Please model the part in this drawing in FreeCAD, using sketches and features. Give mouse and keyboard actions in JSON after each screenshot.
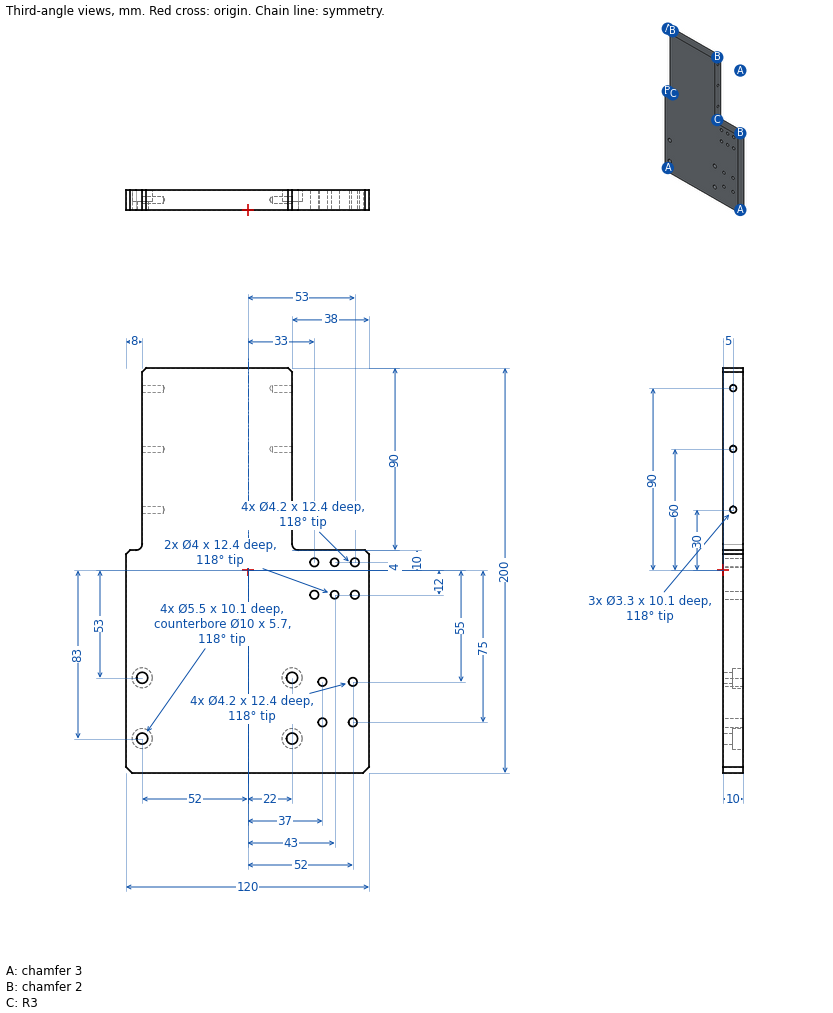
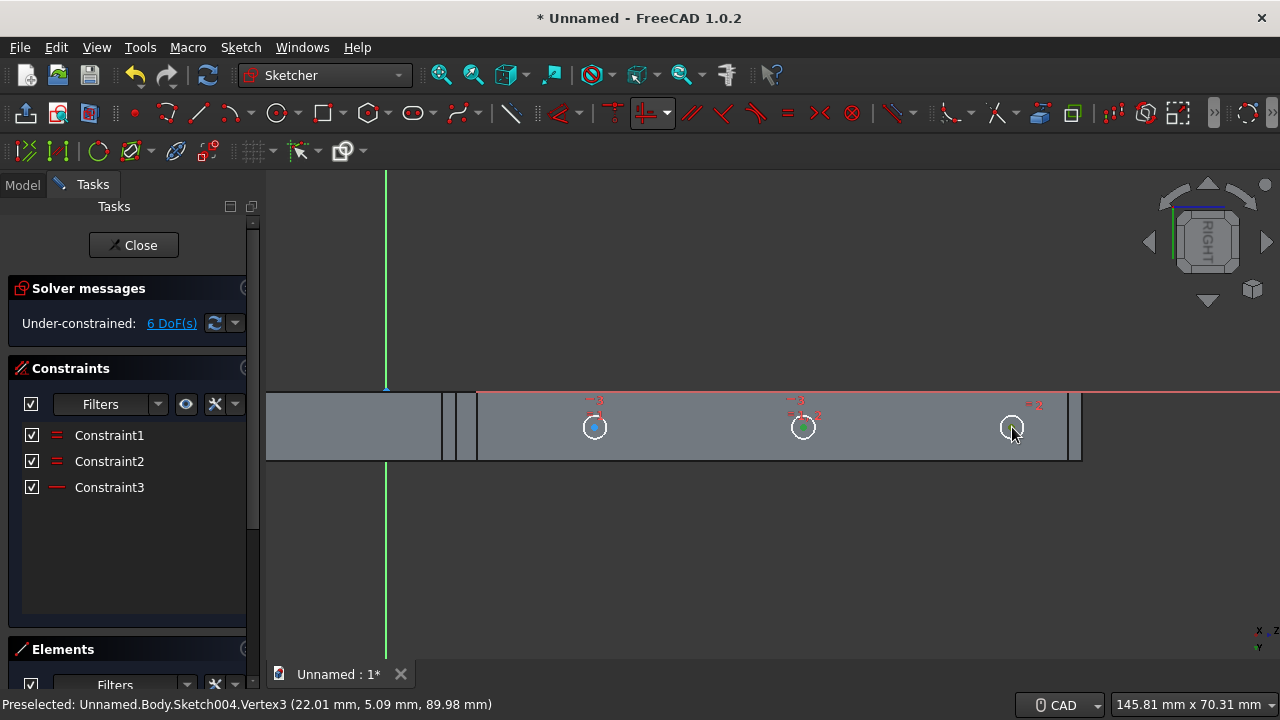
{"action": "key", "text": "h"}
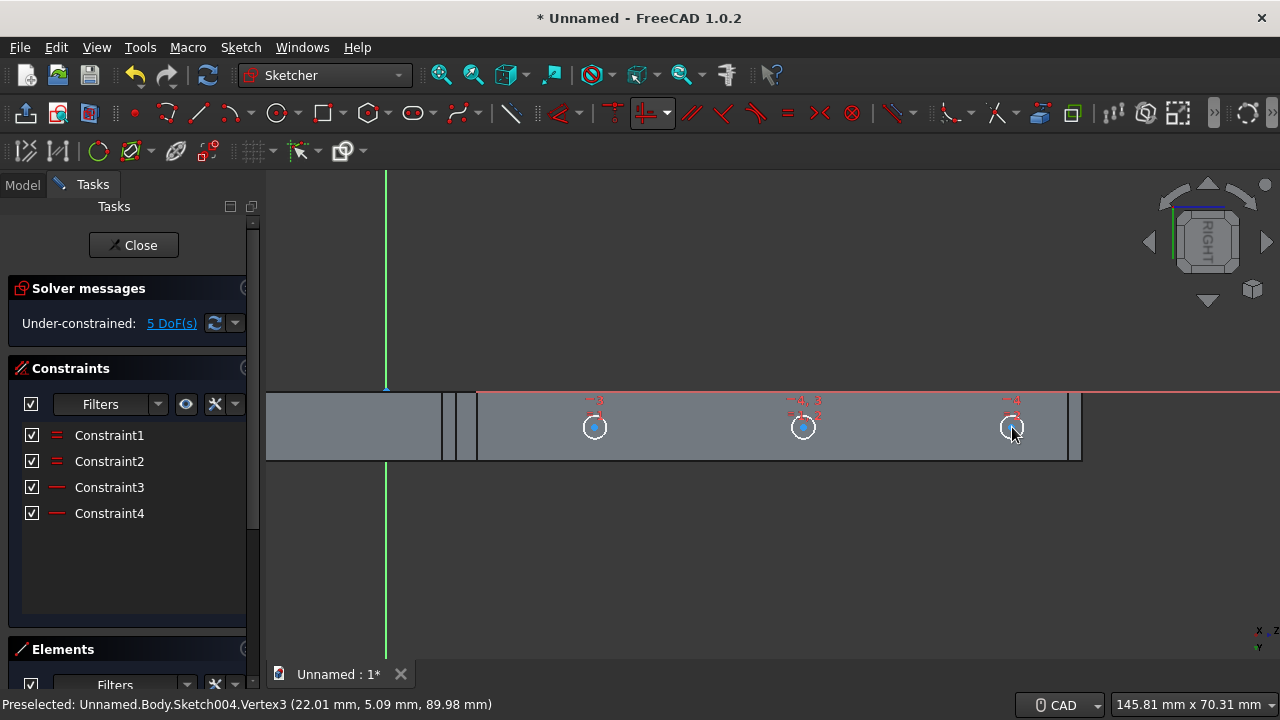
{"action": "left_click", "coordinate": [558, 114]}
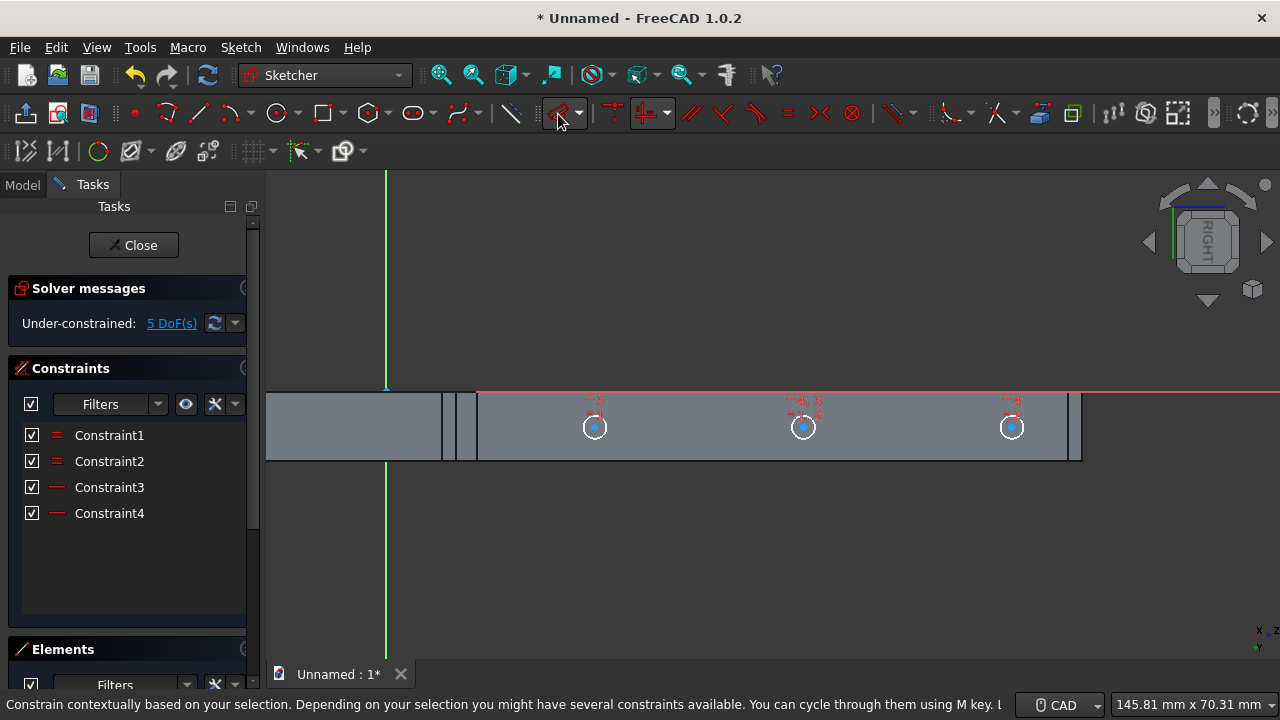
{"action": "scroll", "coordinate": [603, 419], "scroll_direction": "up", "scroll_amount": 3}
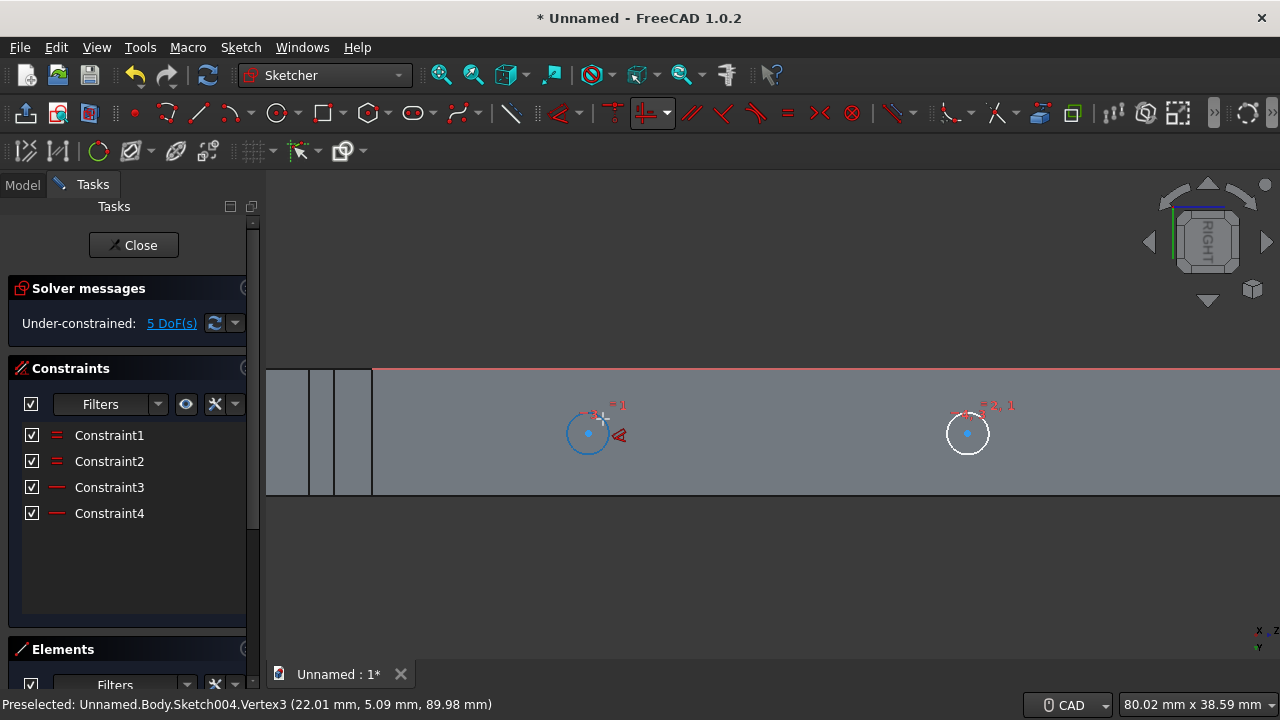
{"action": "left_click", "coordinate": [603, 419]}
{"action": "left_click", "coordinate": [626, 397]}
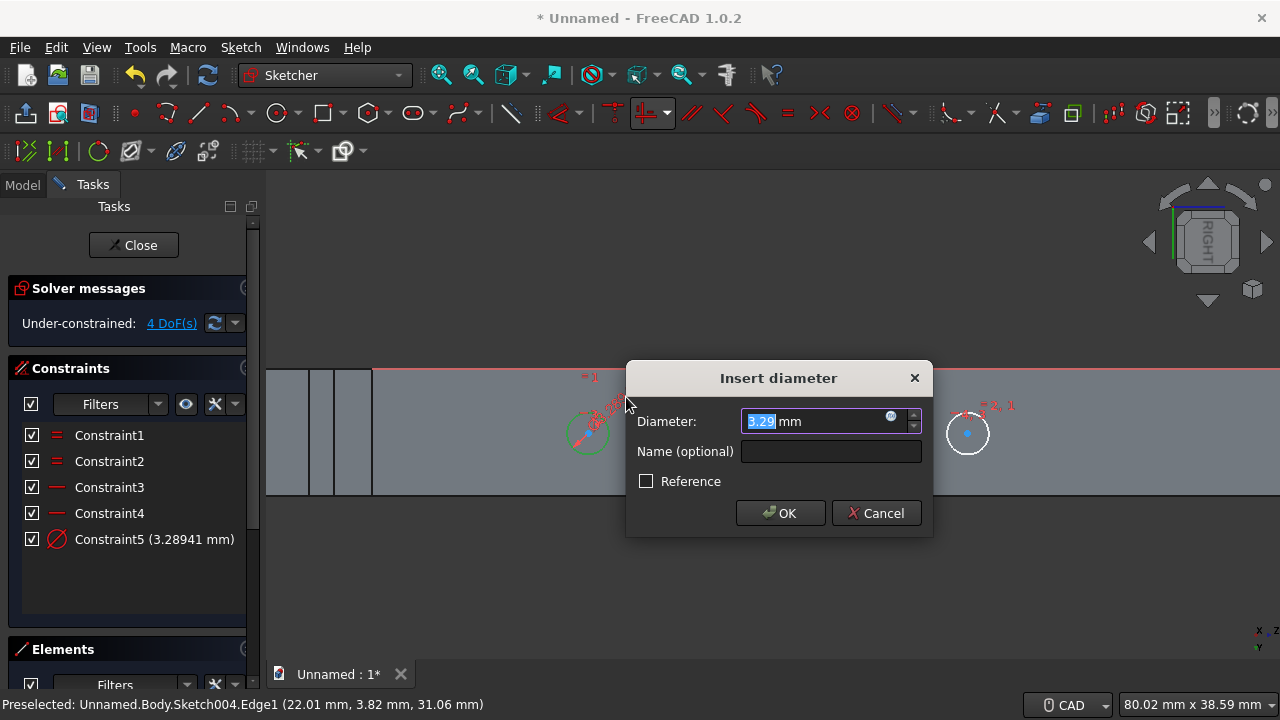
{"action": "type", "text": "3.3"}
{"action": "key", "text": "Return"}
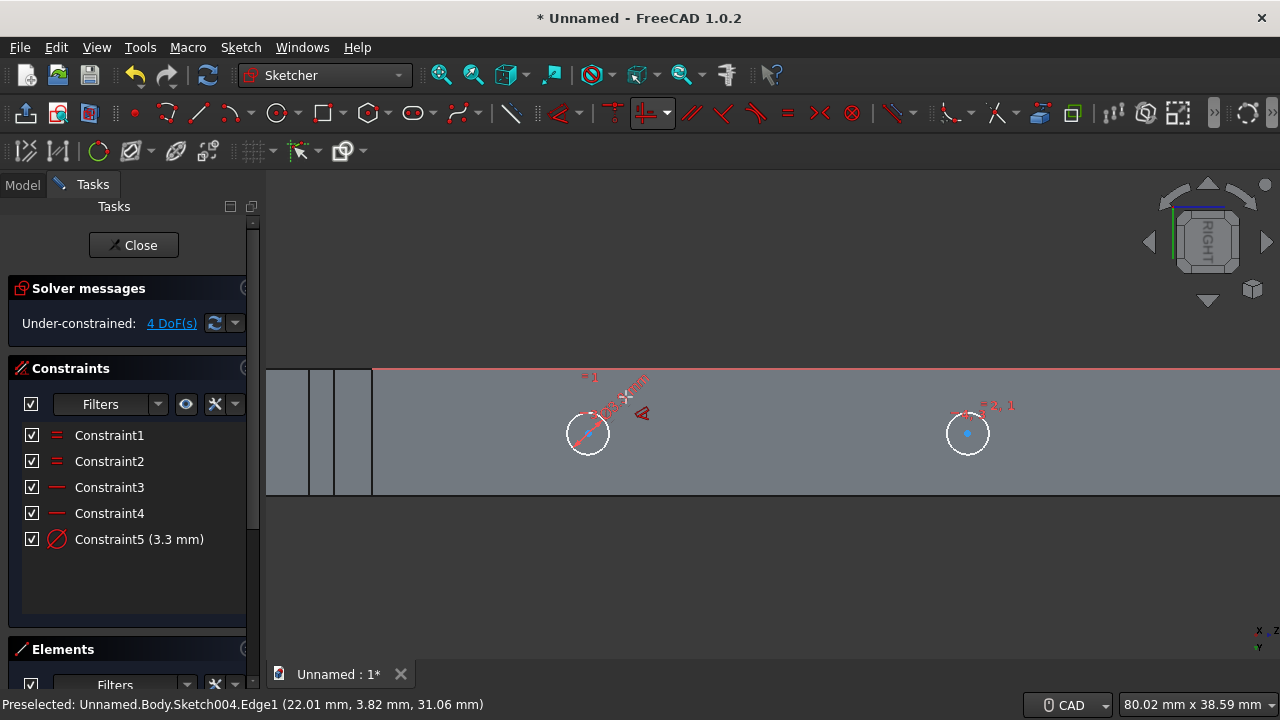
{"action": "left_click", "coordinate": [588, 434]}
{"action": "left_click", "coordinate": [622, 424]}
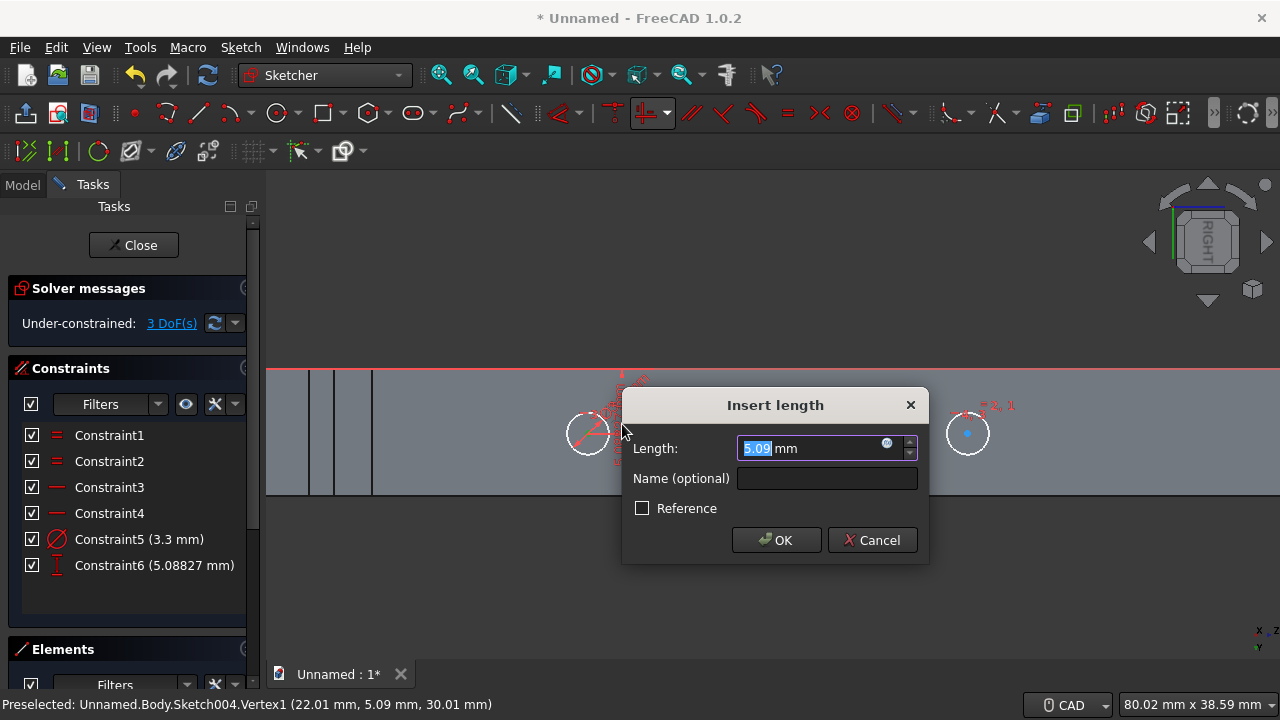
{"action": "type", "text": "5"}
{"action": "key", "text": "Return"}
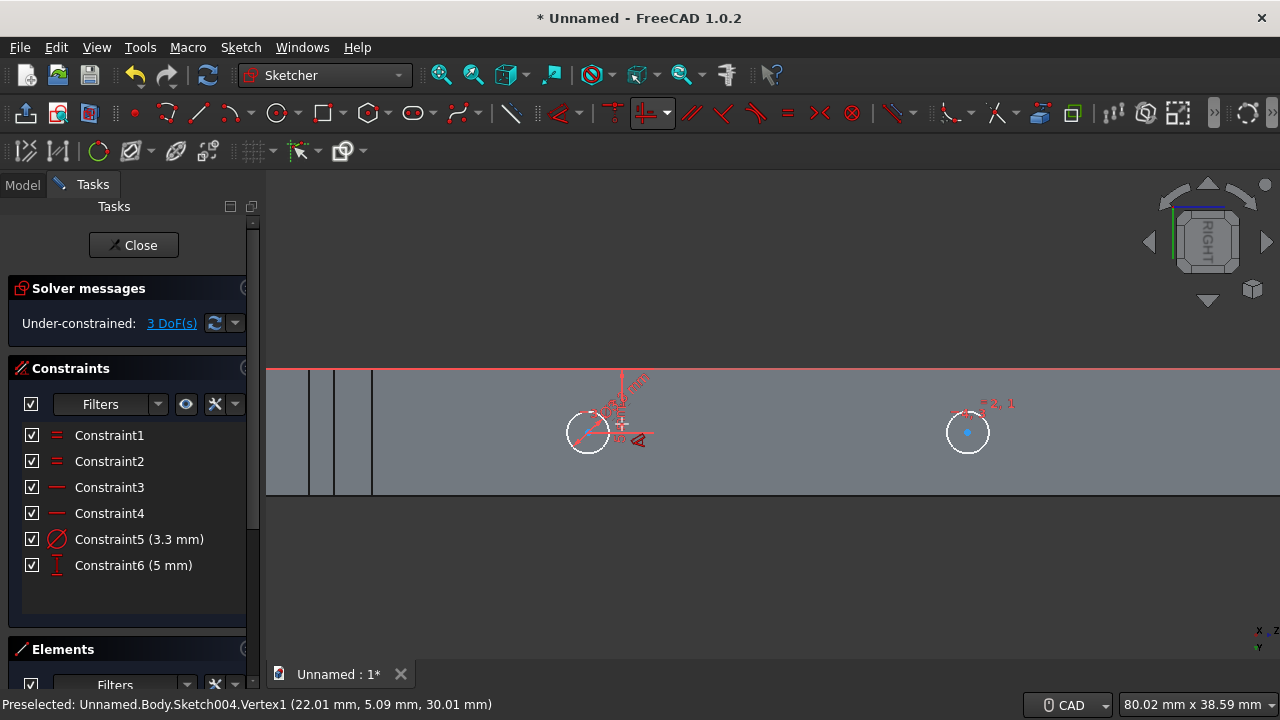
{"action": "left_click", "coordinate": [588, 433]}
{"action": "left_click", "coordinate": [441, 335]}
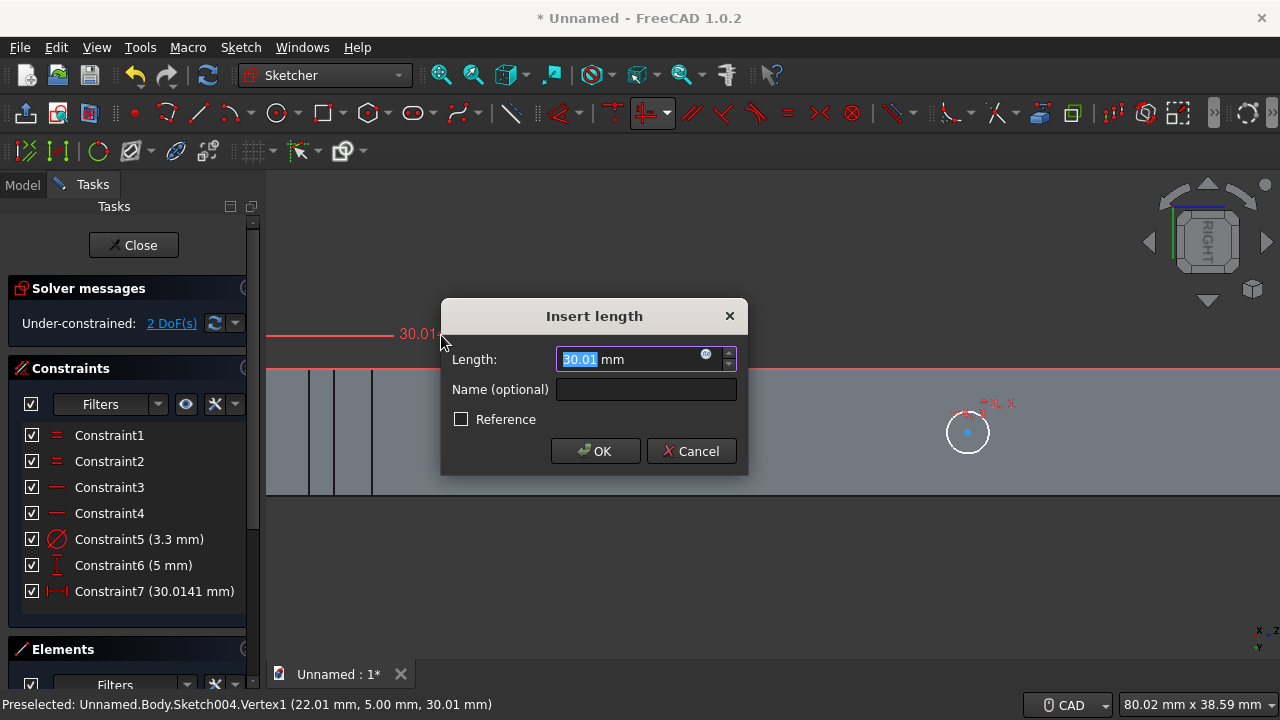
{"action": "type", "text": "30"}
{"action": "key", "text": "Return"}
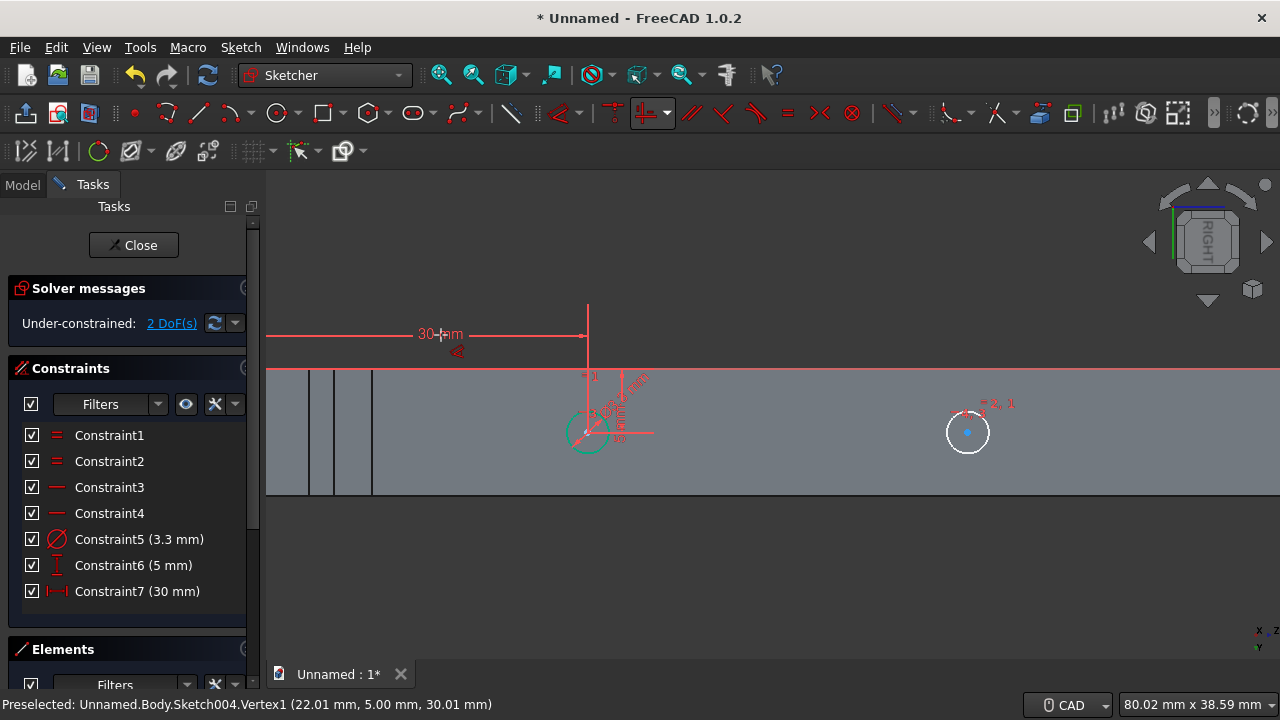
{"action": "left_click", "coordinate": [968, 433]}
{"action": "left_click", "coordinate": [631, 335]}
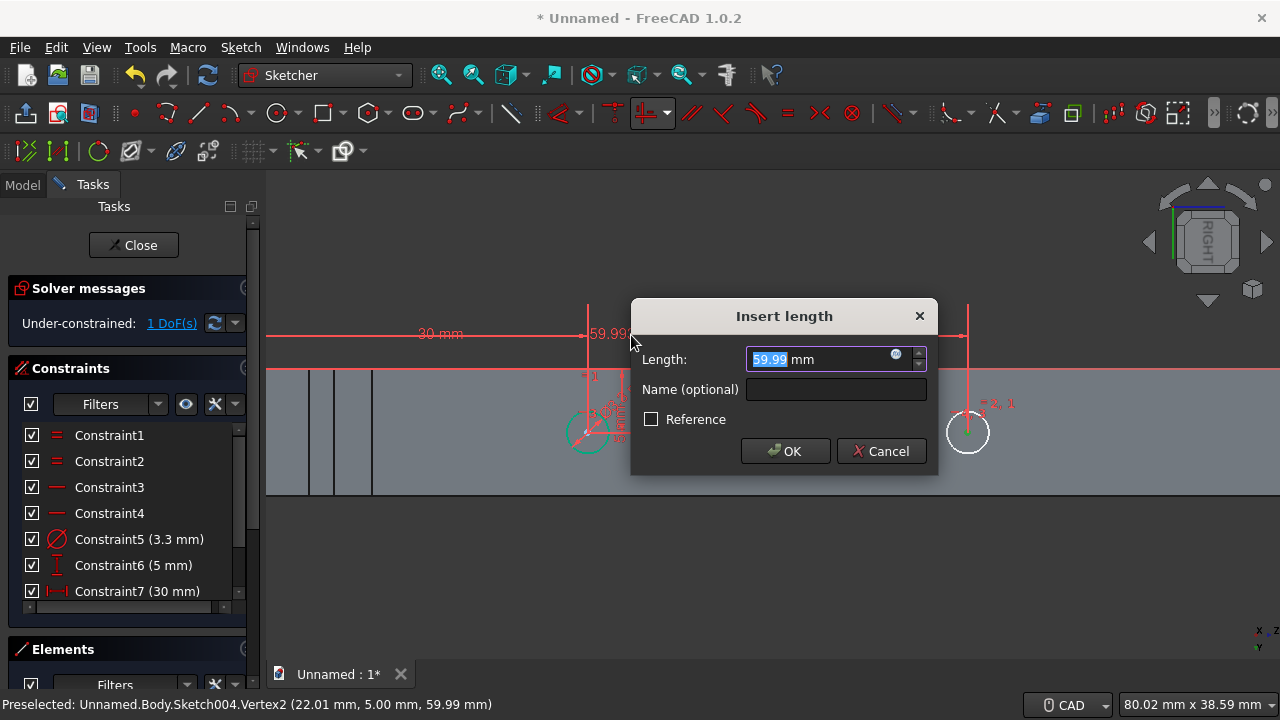
{"action": "type", "text": "60"}
{"action": "key", "text": "Return"}